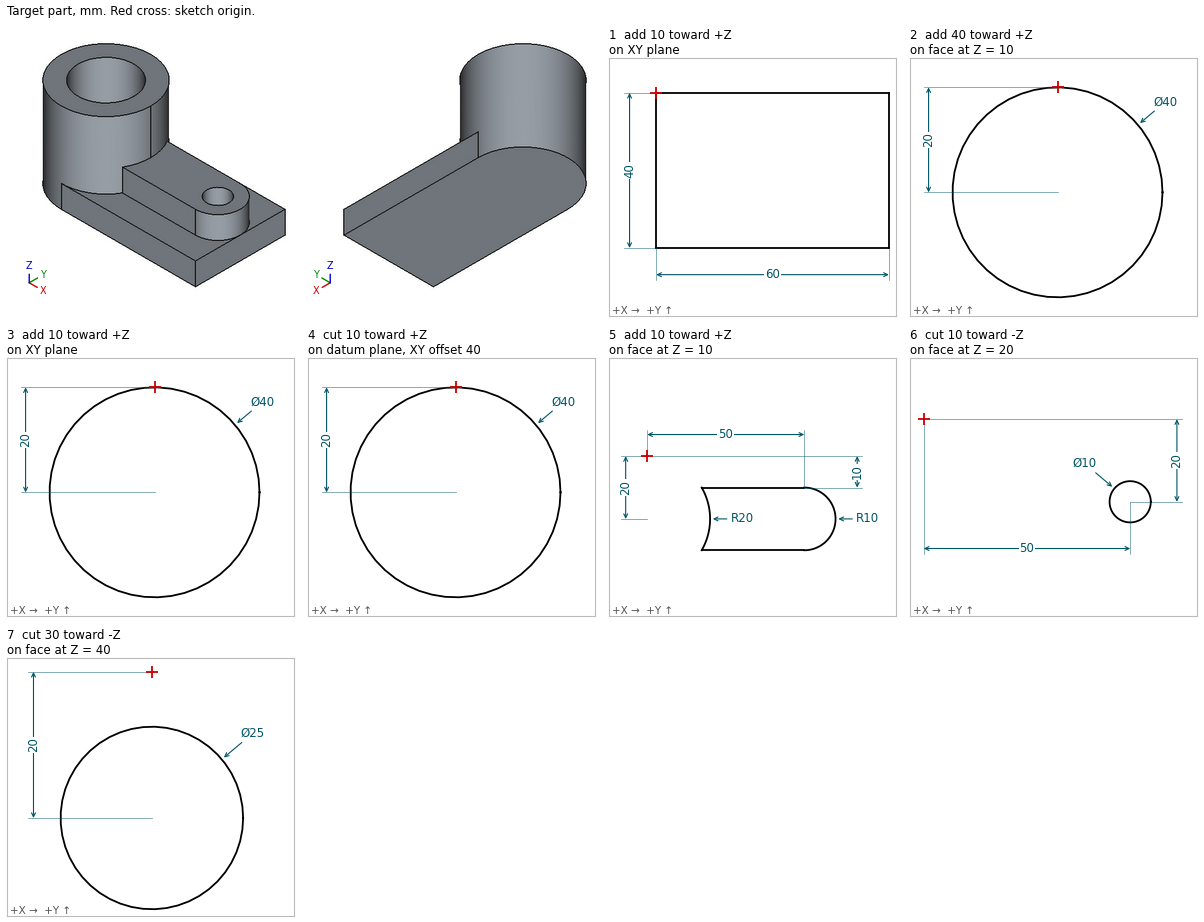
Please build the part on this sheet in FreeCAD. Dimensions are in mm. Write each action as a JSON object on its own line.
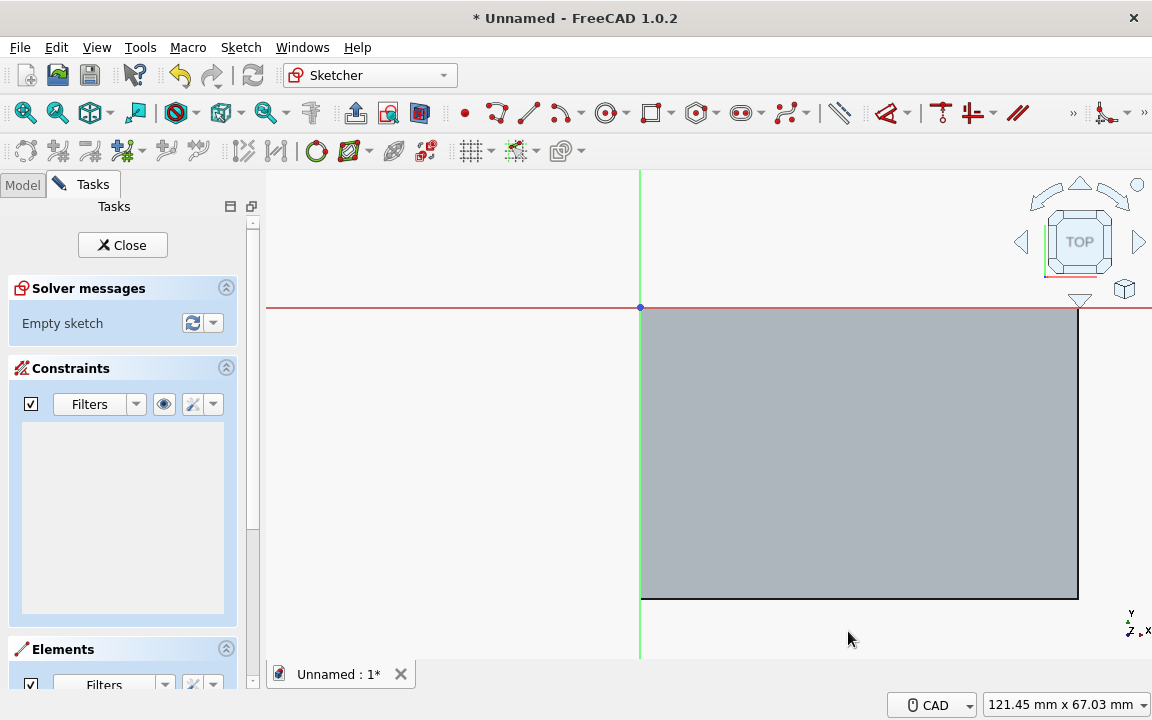
{"action": "left_click", "coordinate": [606, 114]}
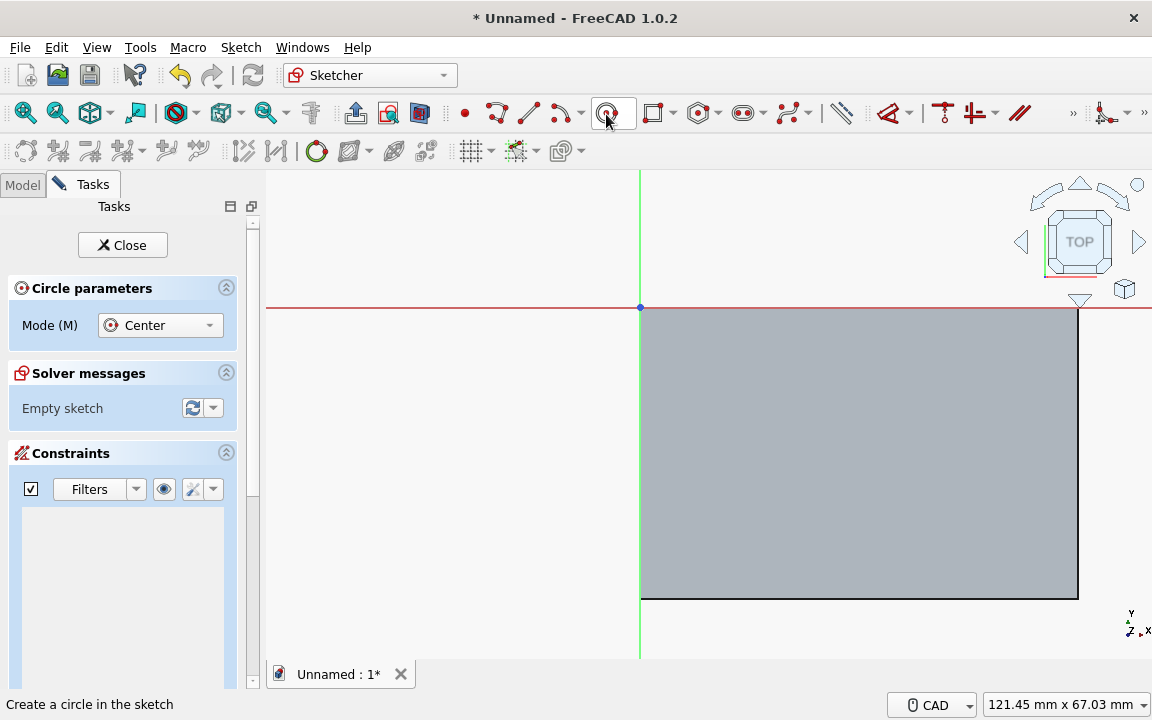
{"action": "left_click", "coordinate": [640, 453]}
{"action": "left_click", "coordinate": [743, 350]}
{"action": "key", "text": "Escape"}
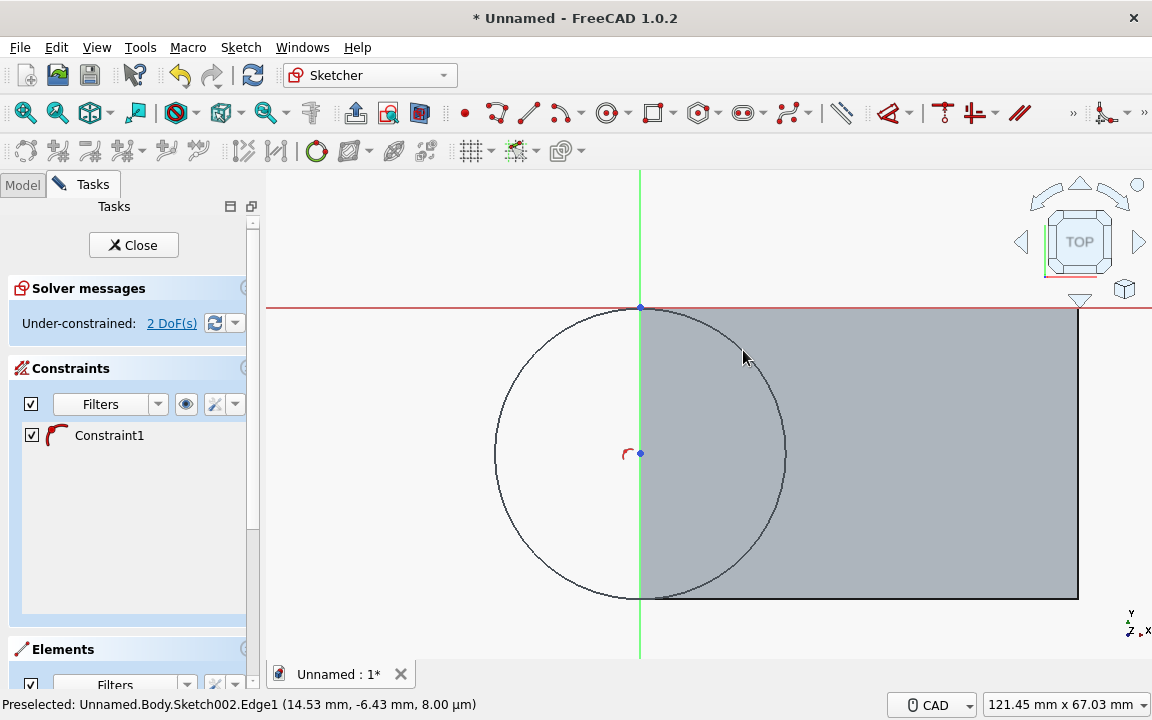
{"action": "left_click", "coordinate": [888, 114]}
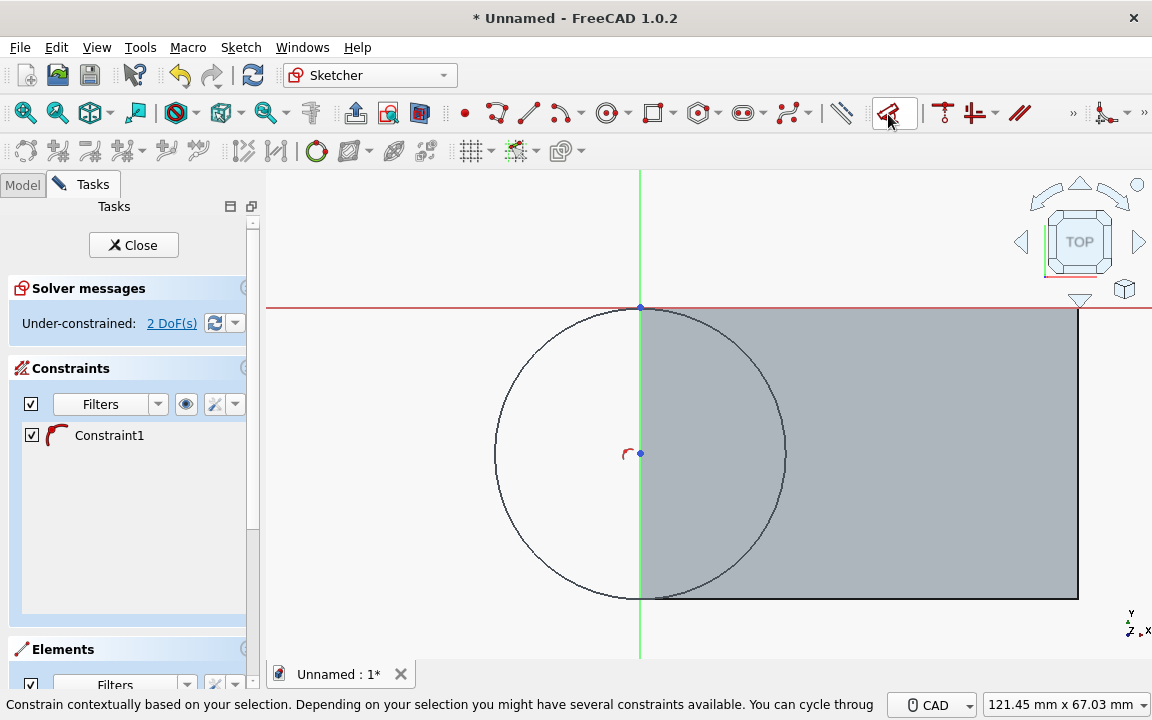
{"action": "left_click", "coordinate": [743, 351]}
{"action": "left_click", "coordinate": [766, 328]}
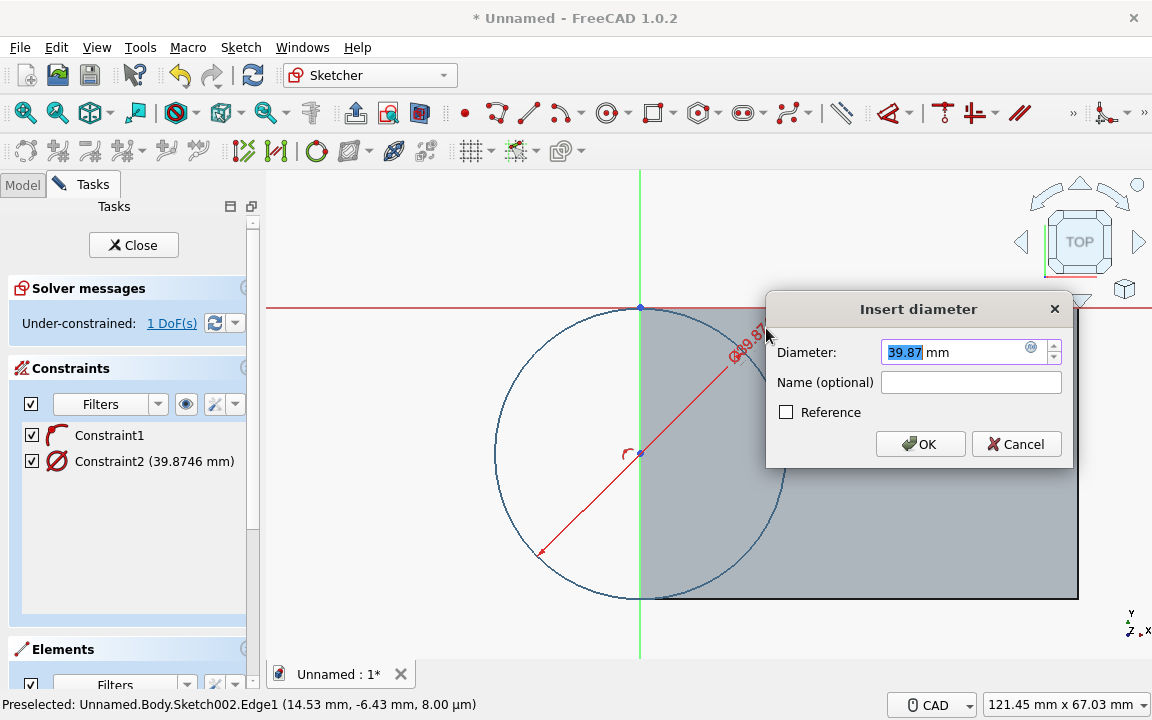
{"action": "type", "text": "40"}
{"action": "key", "text": "Return"}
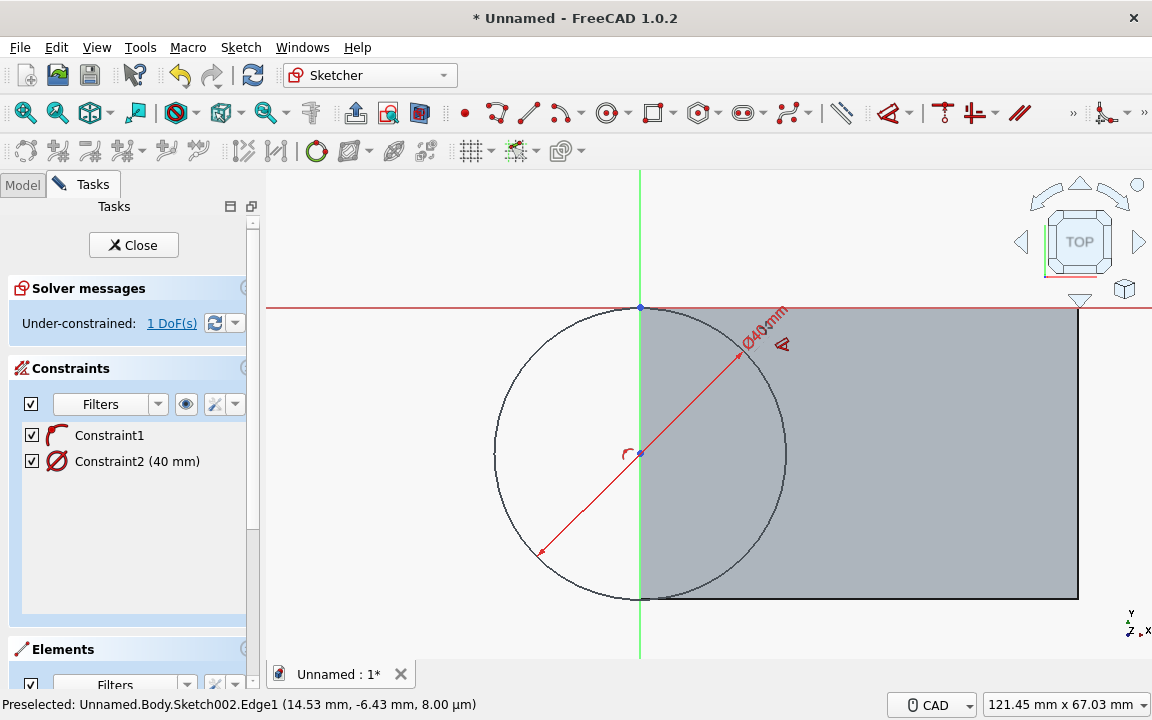
{"action": "left_click", "coordinate": [640, 454]}
{"action": "left_click", "coordinate": [674, 381]}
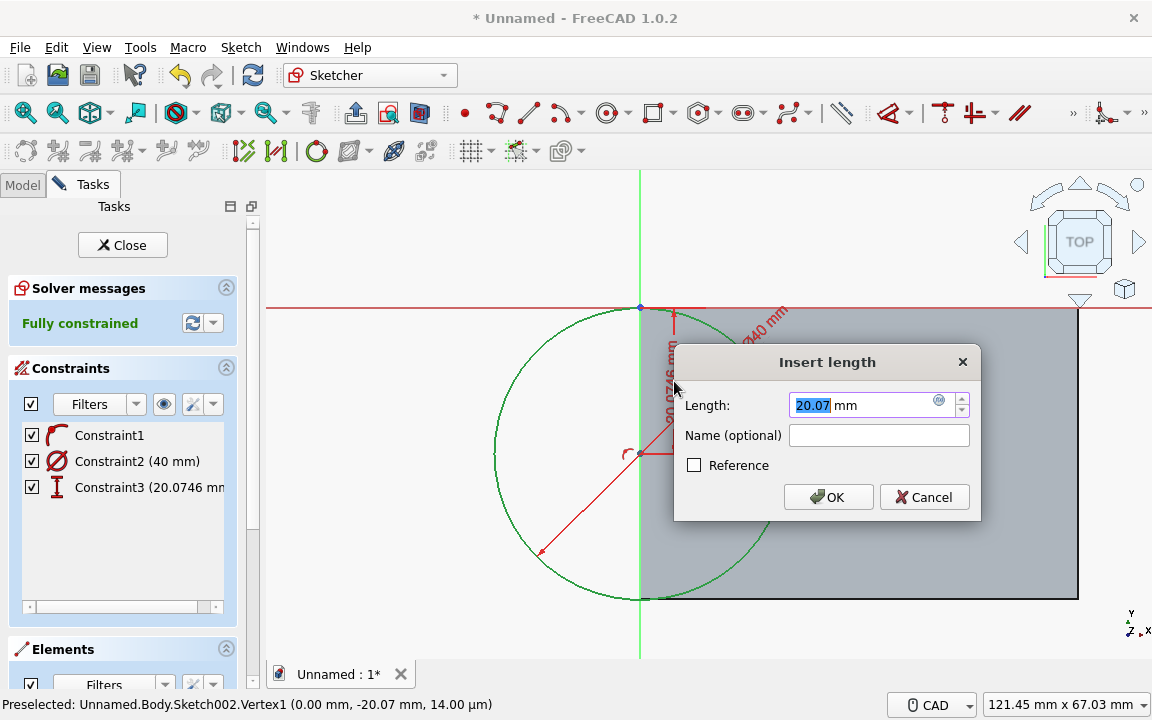
{"action": "type", "text": "20"}
{"action": "key", "text": "Return"}
{"action": "key", "text": "Escape"}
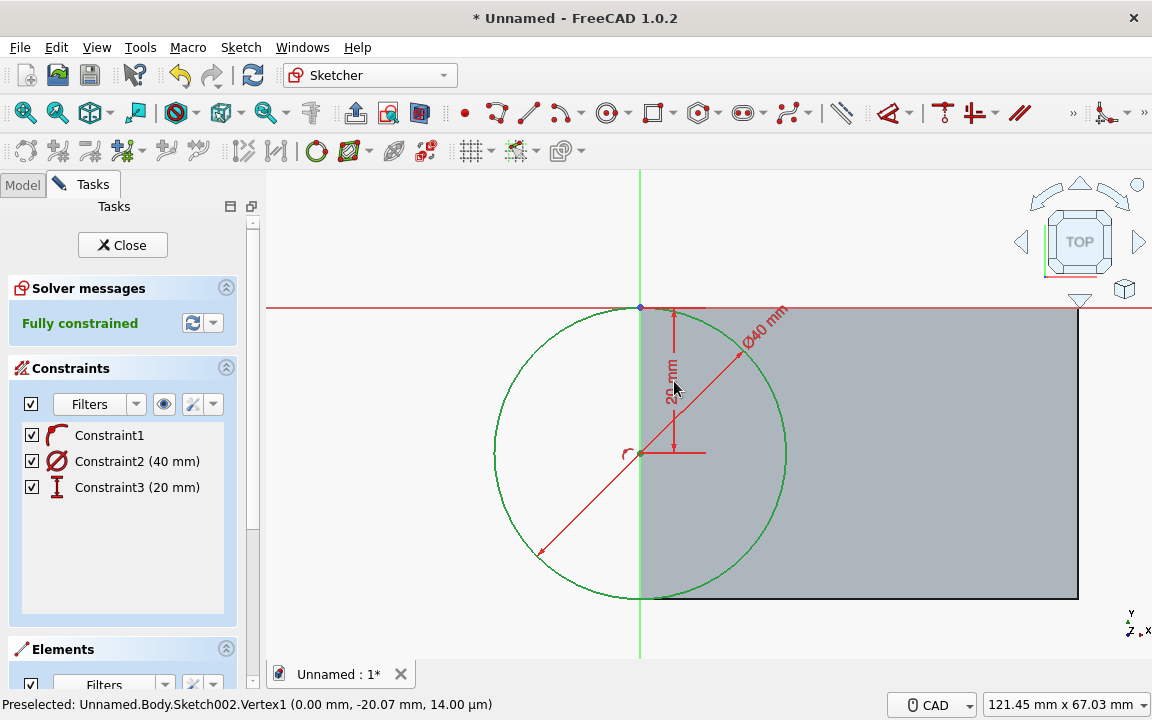
{"action": "left_click", "coordinate": [123, 245]}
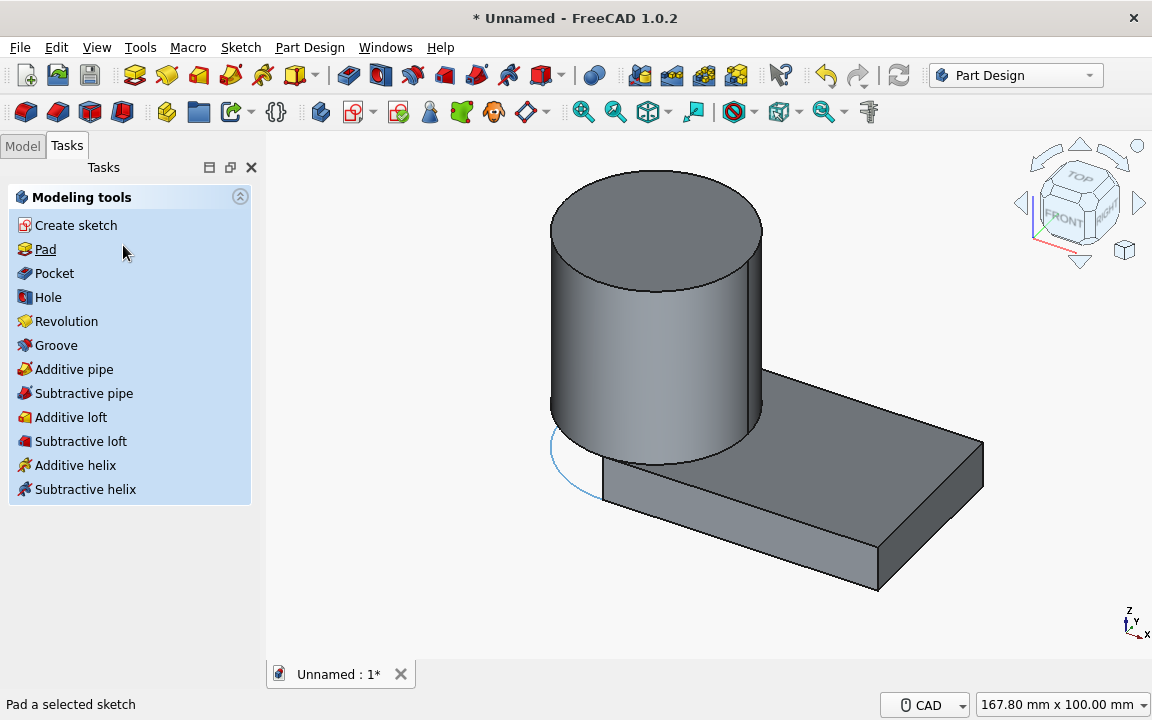
{"action": "left_click", "coordinate": [136, 76]}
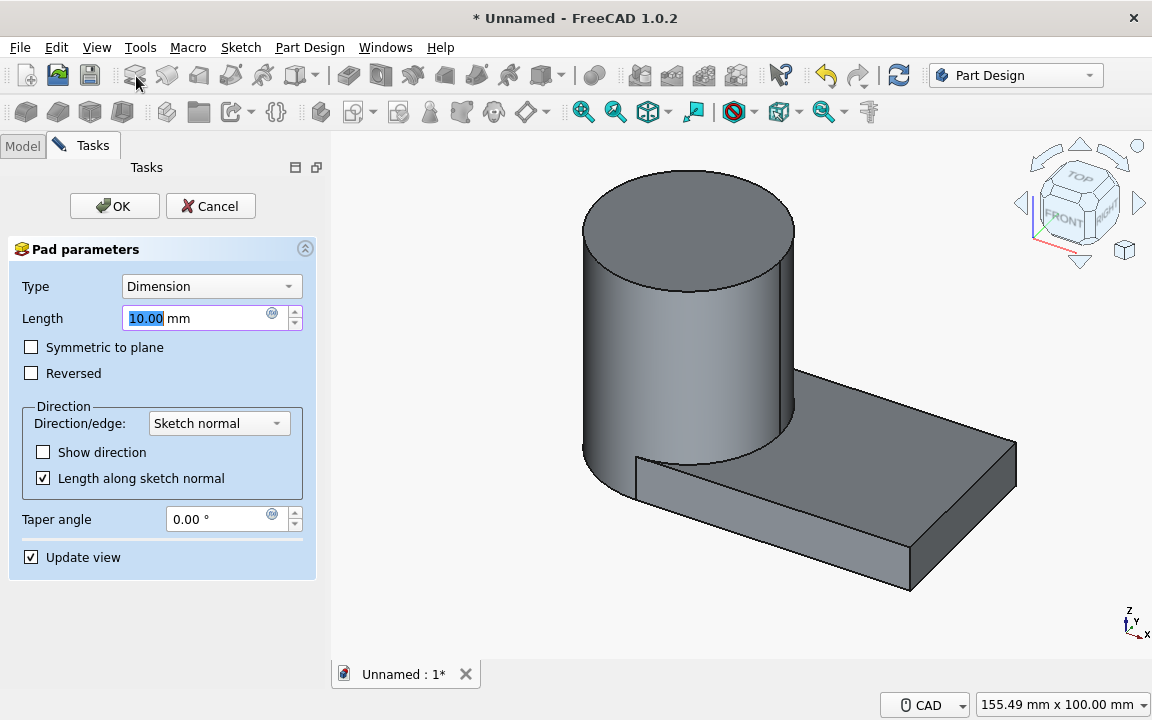
{"action": "type", "text": "10"}
{"action": "key", "text": "Tab"}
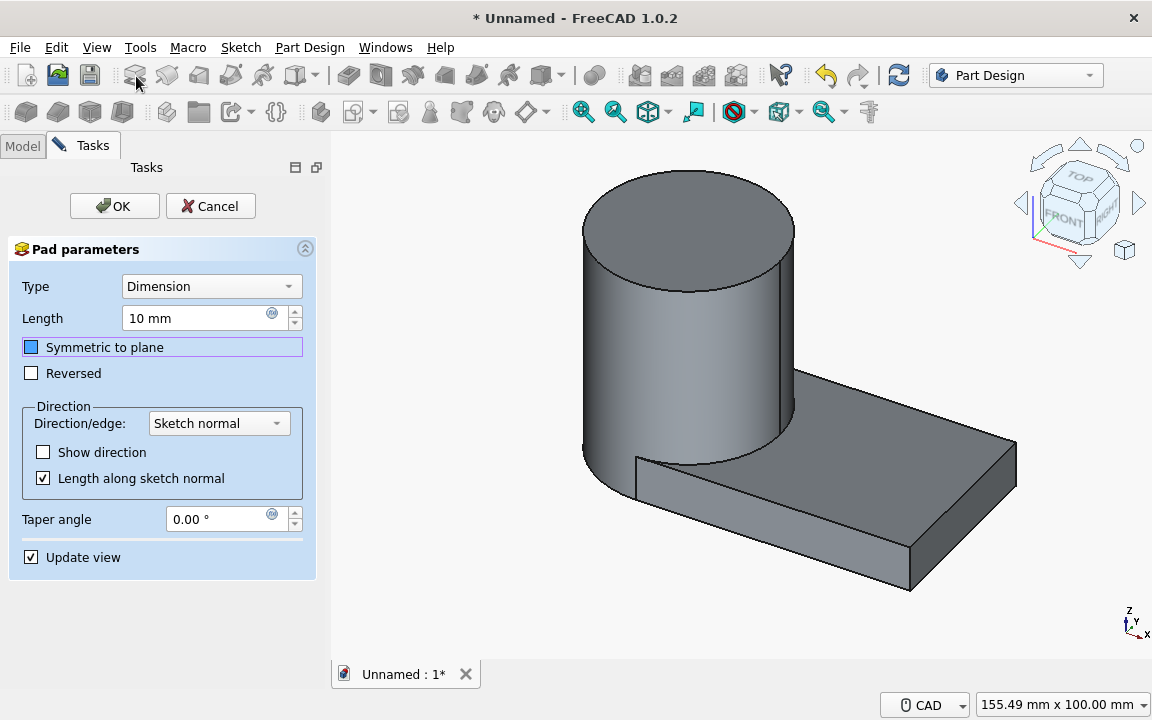
{"action": "left_click", "coordinate": [115, 206]}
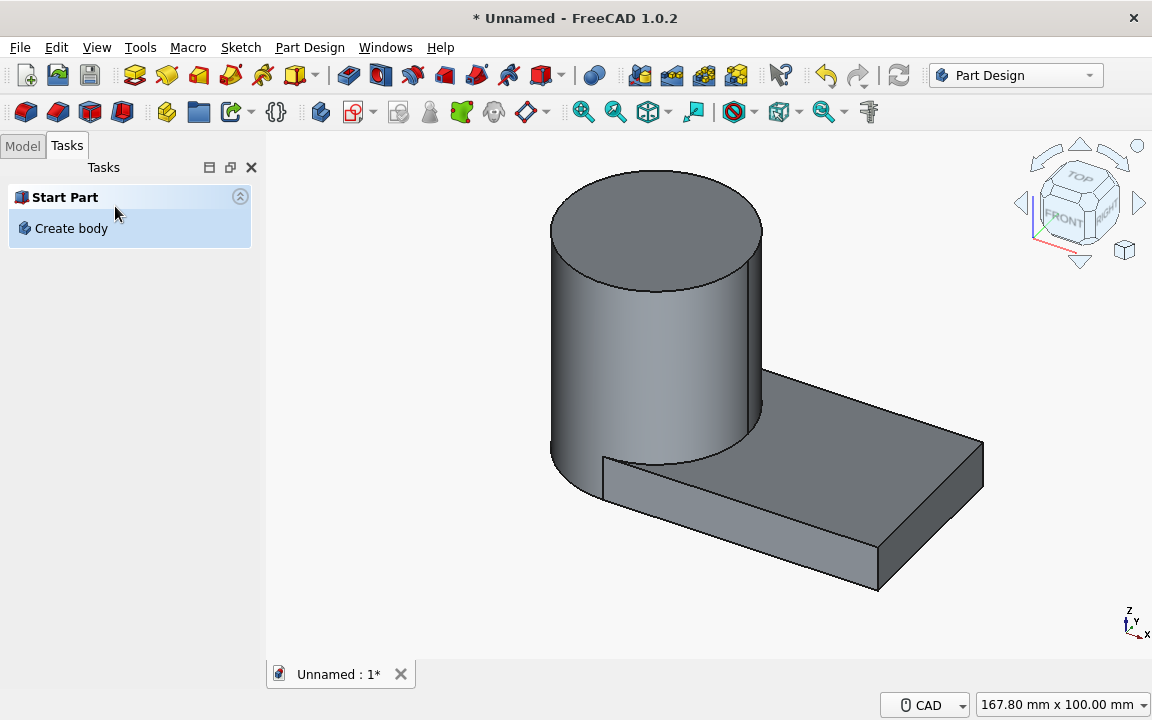
{"action": "left_click", "coordinate": [23, 145]}